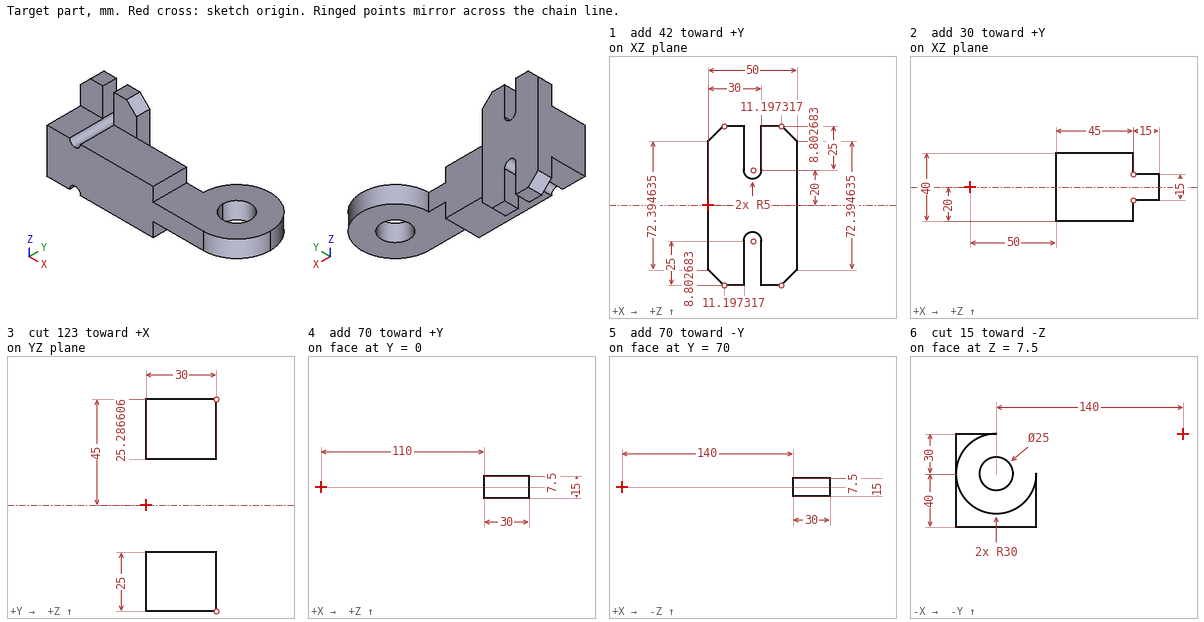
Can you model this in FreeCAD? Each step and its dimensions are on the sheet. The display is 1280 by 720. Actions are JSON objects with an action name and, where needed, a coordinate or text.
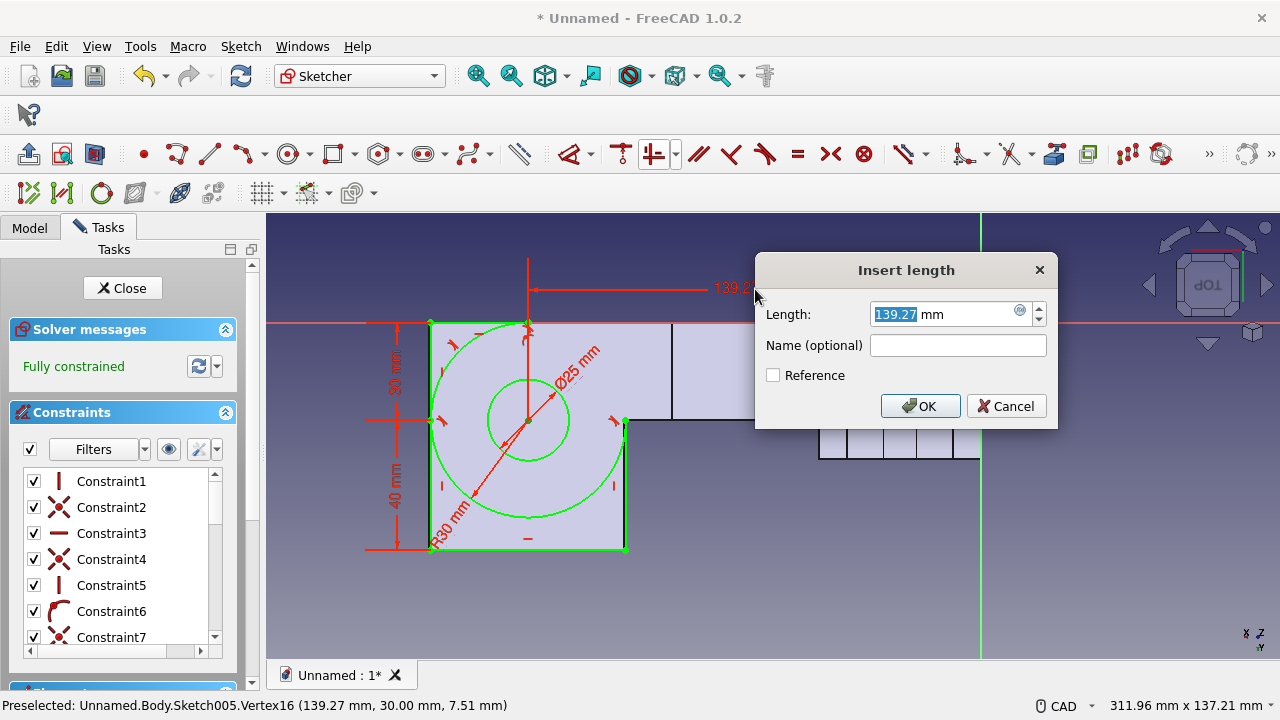
{"action": "type", "text": "140"}
{"action": "key", "text": "Return"}
{"action": "key", "text": "Escape"}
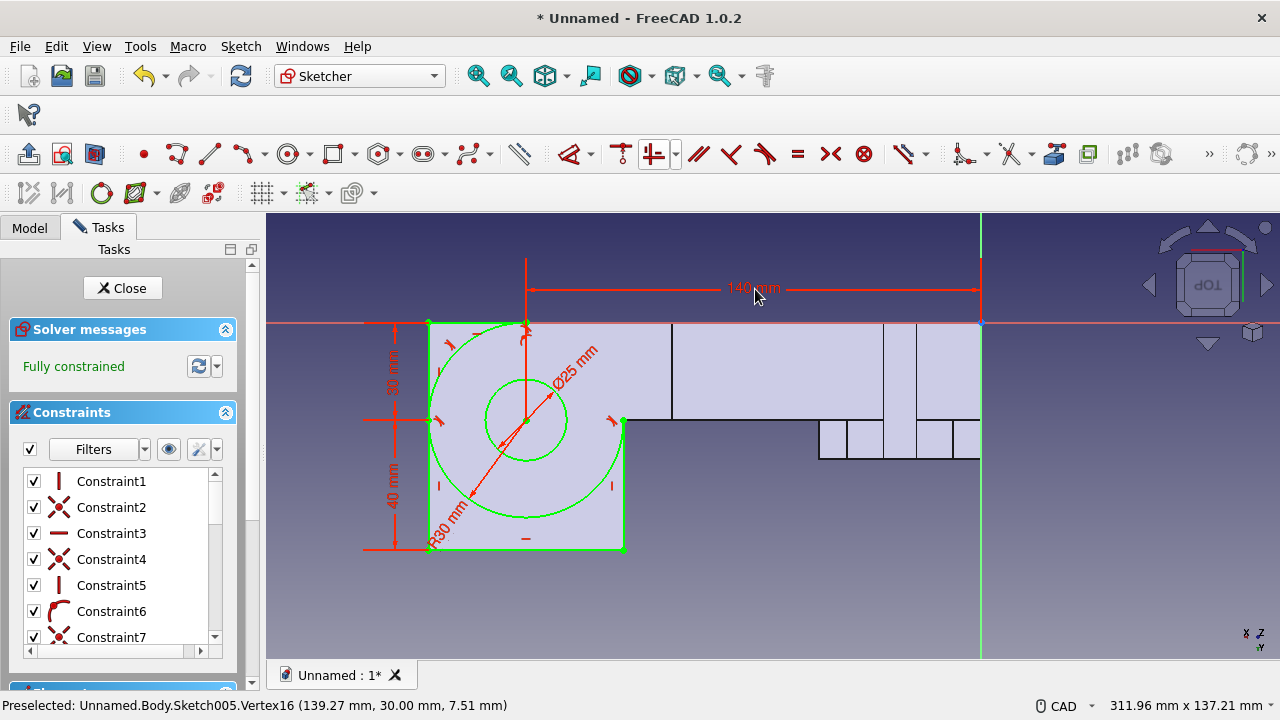
{"action": "left_click", "coordinate": [123, 288]}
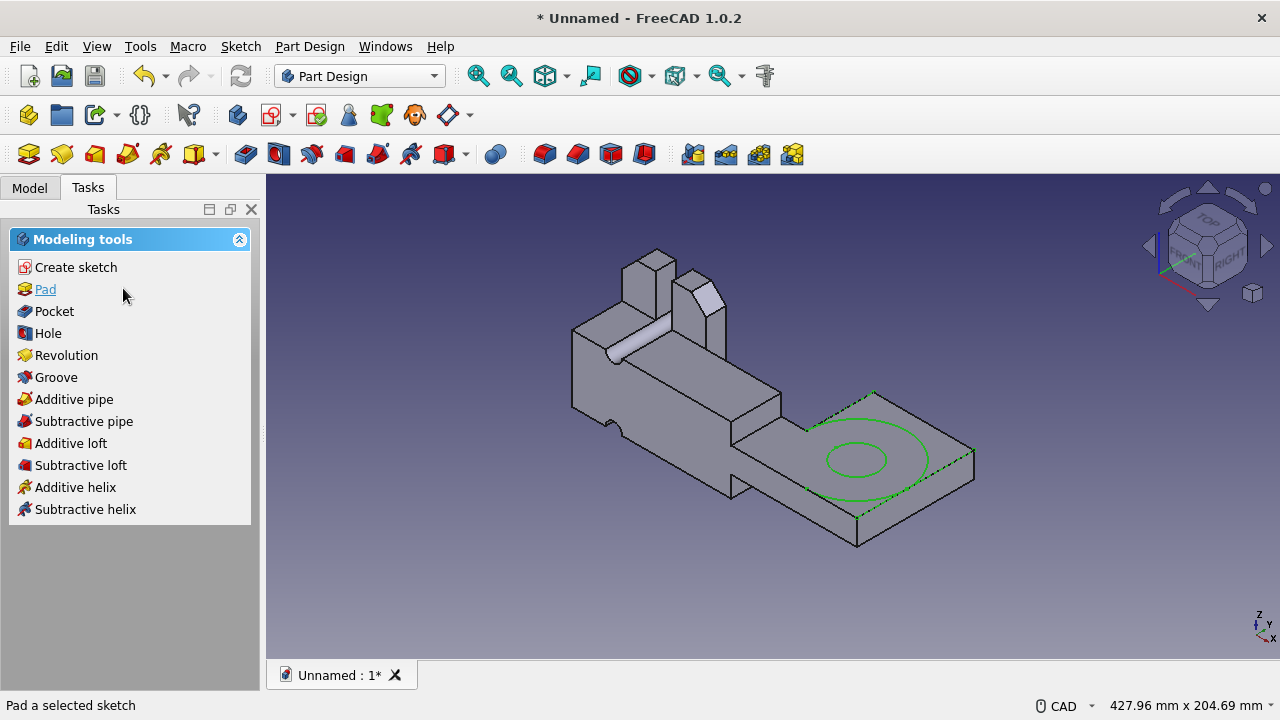
{"action": "left_click", "coordinate": [246, 154]}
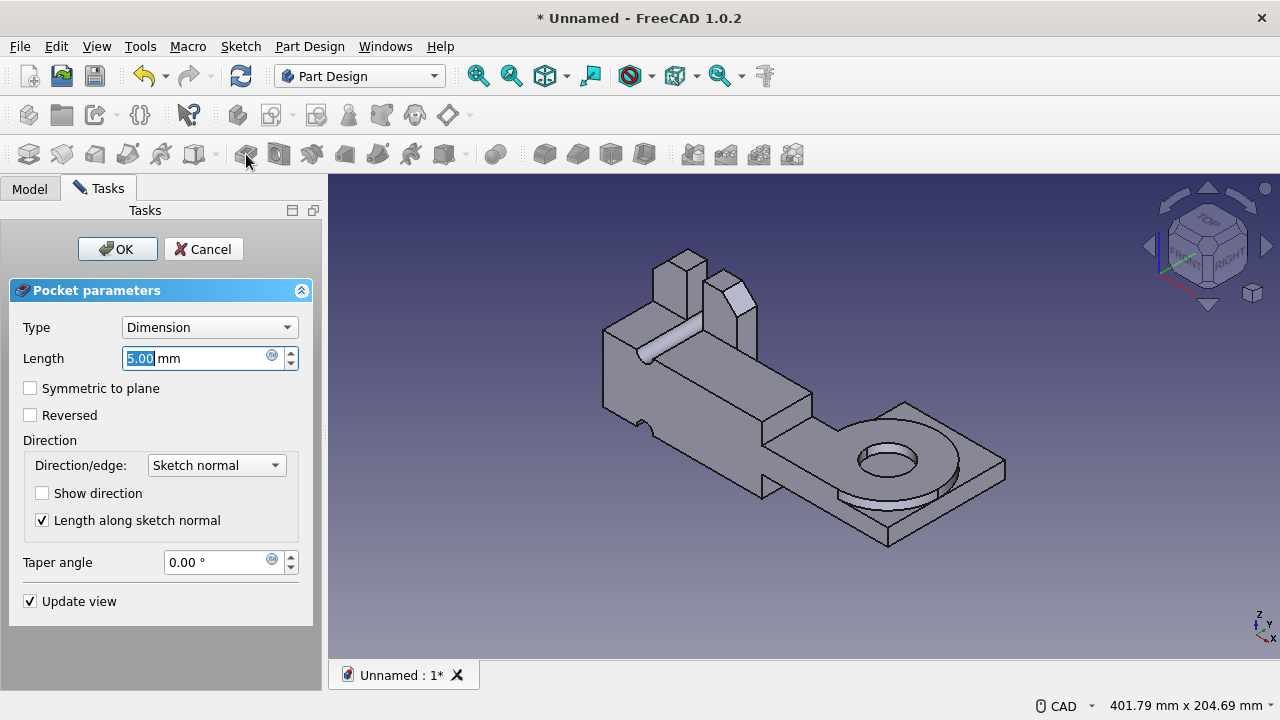
{"action": "type", "text": "15"}
{"action": "key", "text": "Tab"}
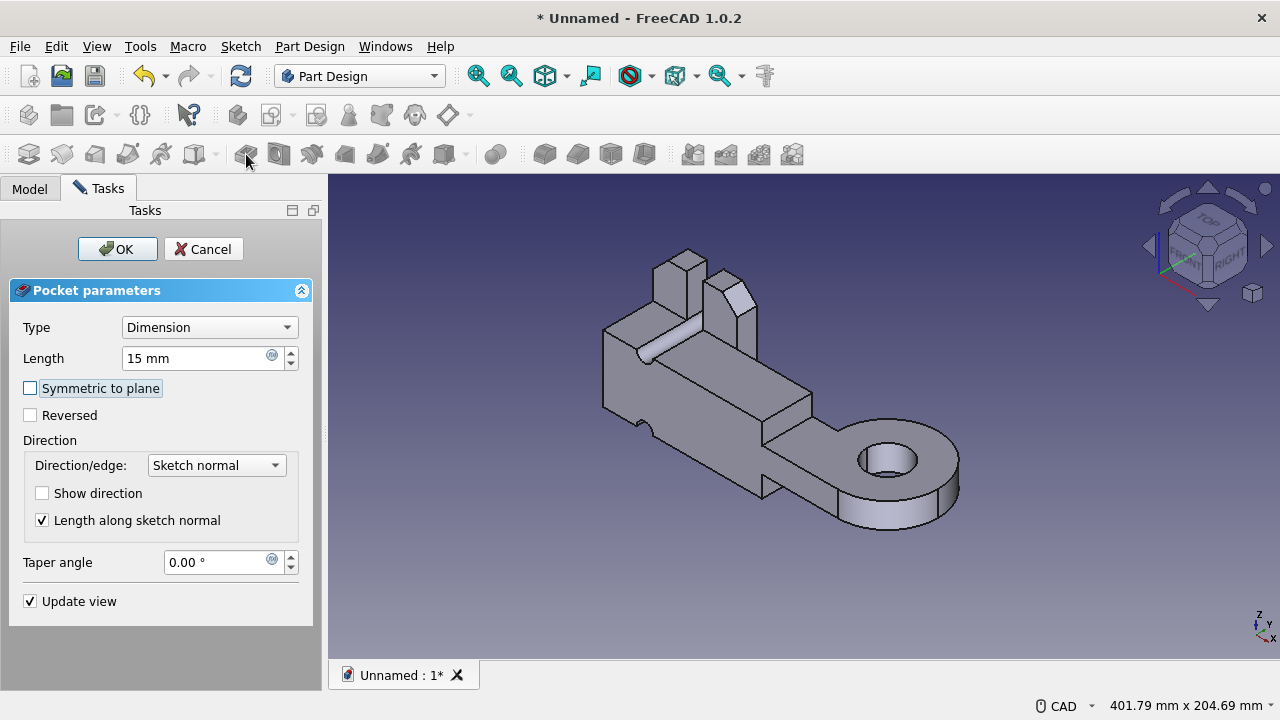
{"action": "left_click", "coordinate": [118, 249]}